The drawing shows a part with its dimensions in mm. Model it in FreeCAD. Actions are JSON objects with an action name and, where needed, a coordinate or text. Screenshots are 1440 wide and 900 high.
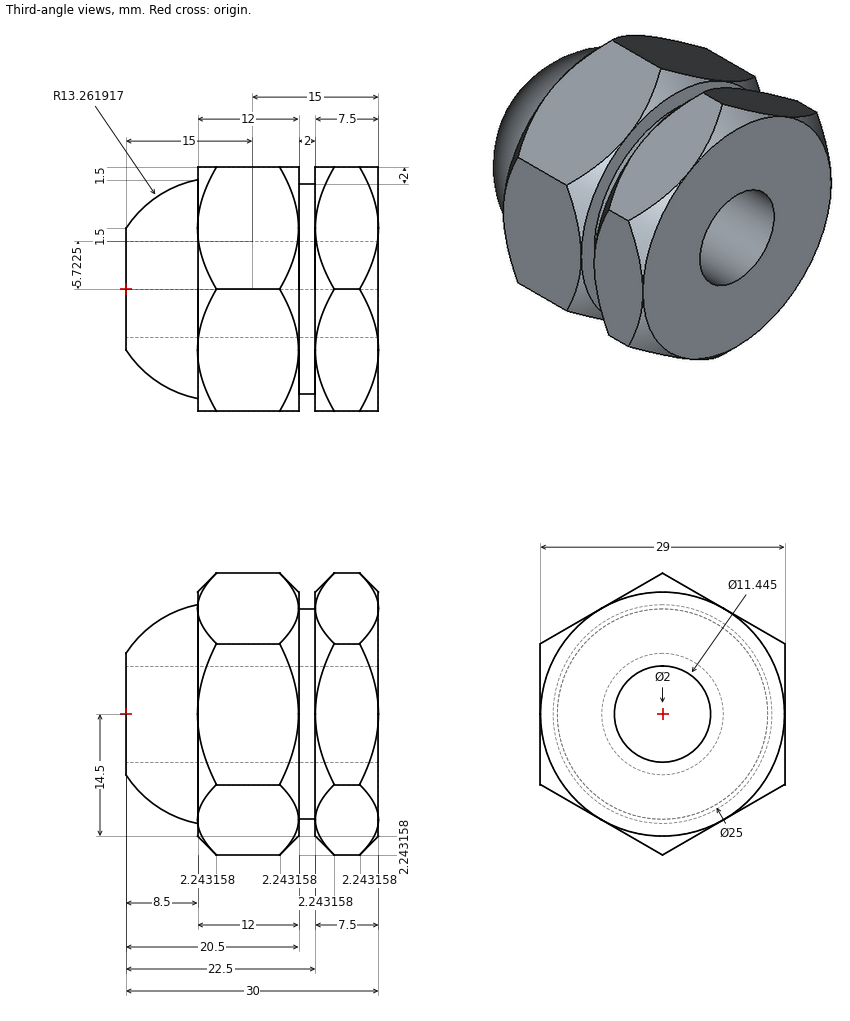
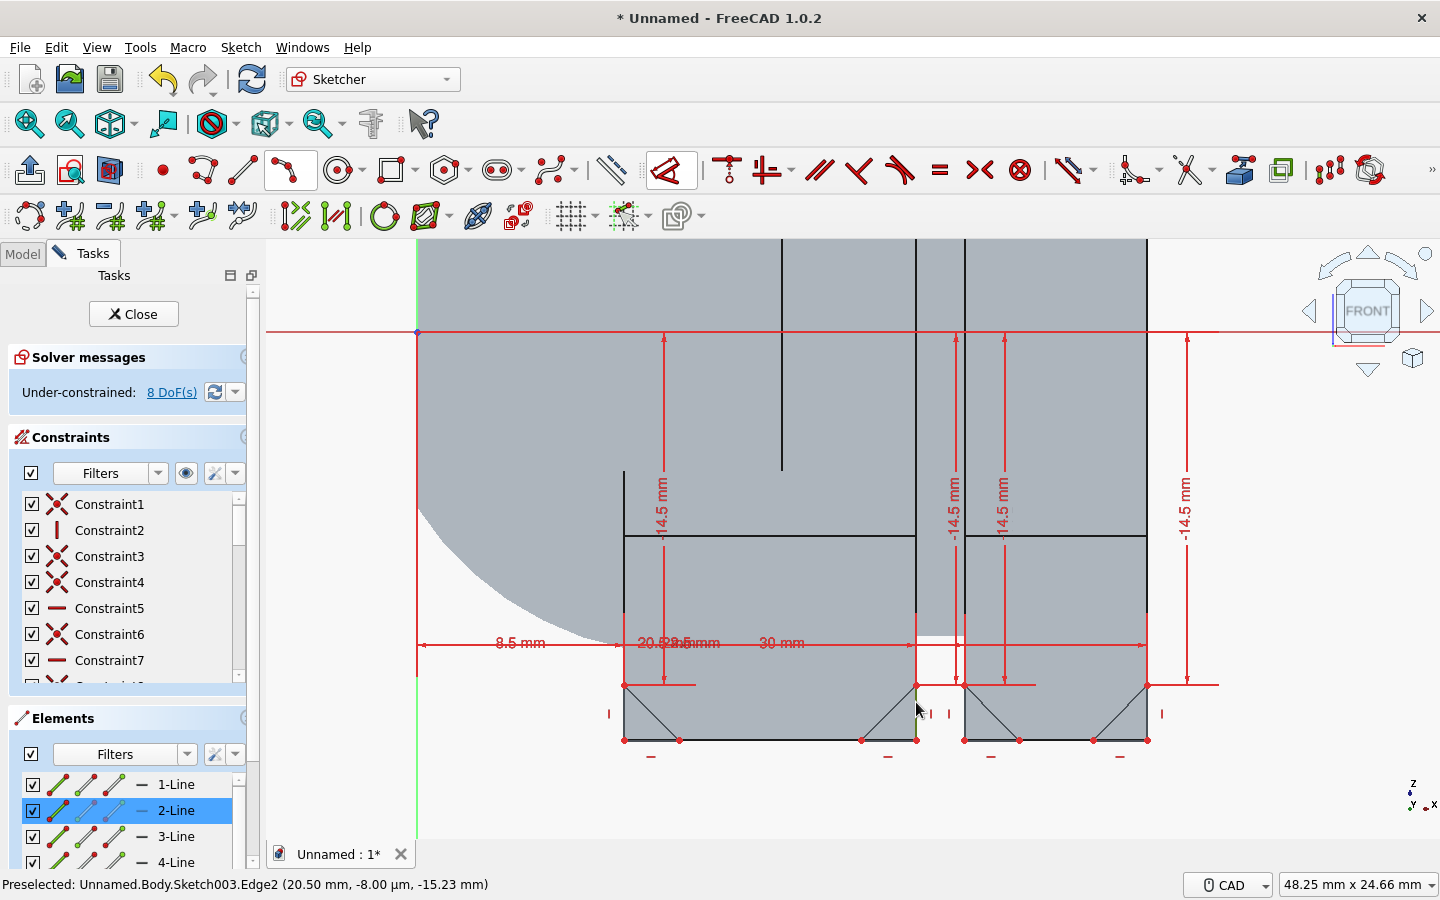
{"action": "key", "text": "i"}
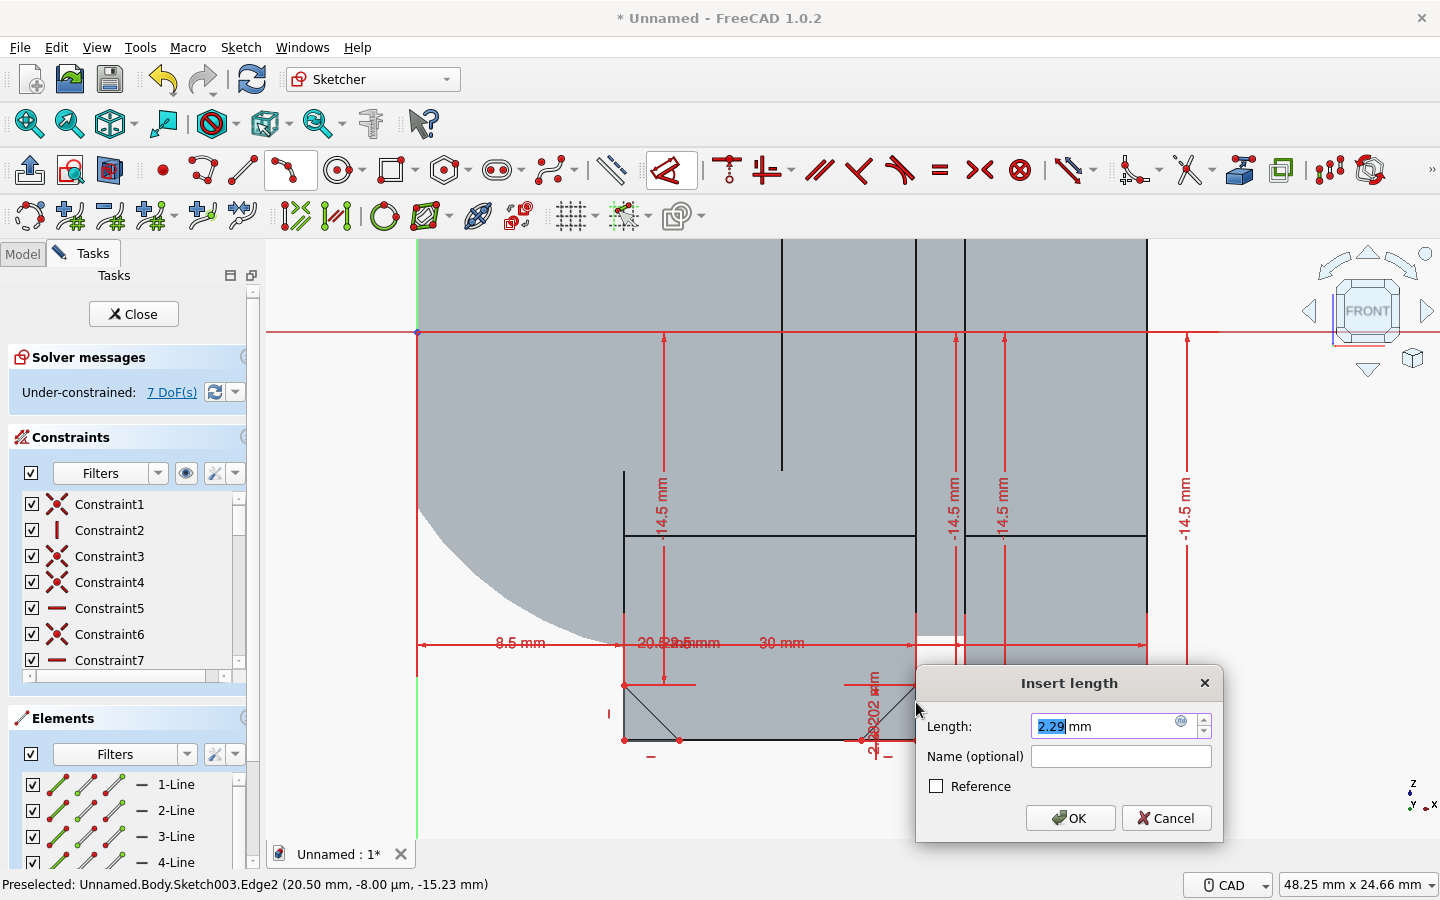
{"action": "type", "text": "2.243158"}
{"action": "key", "text": "Return"}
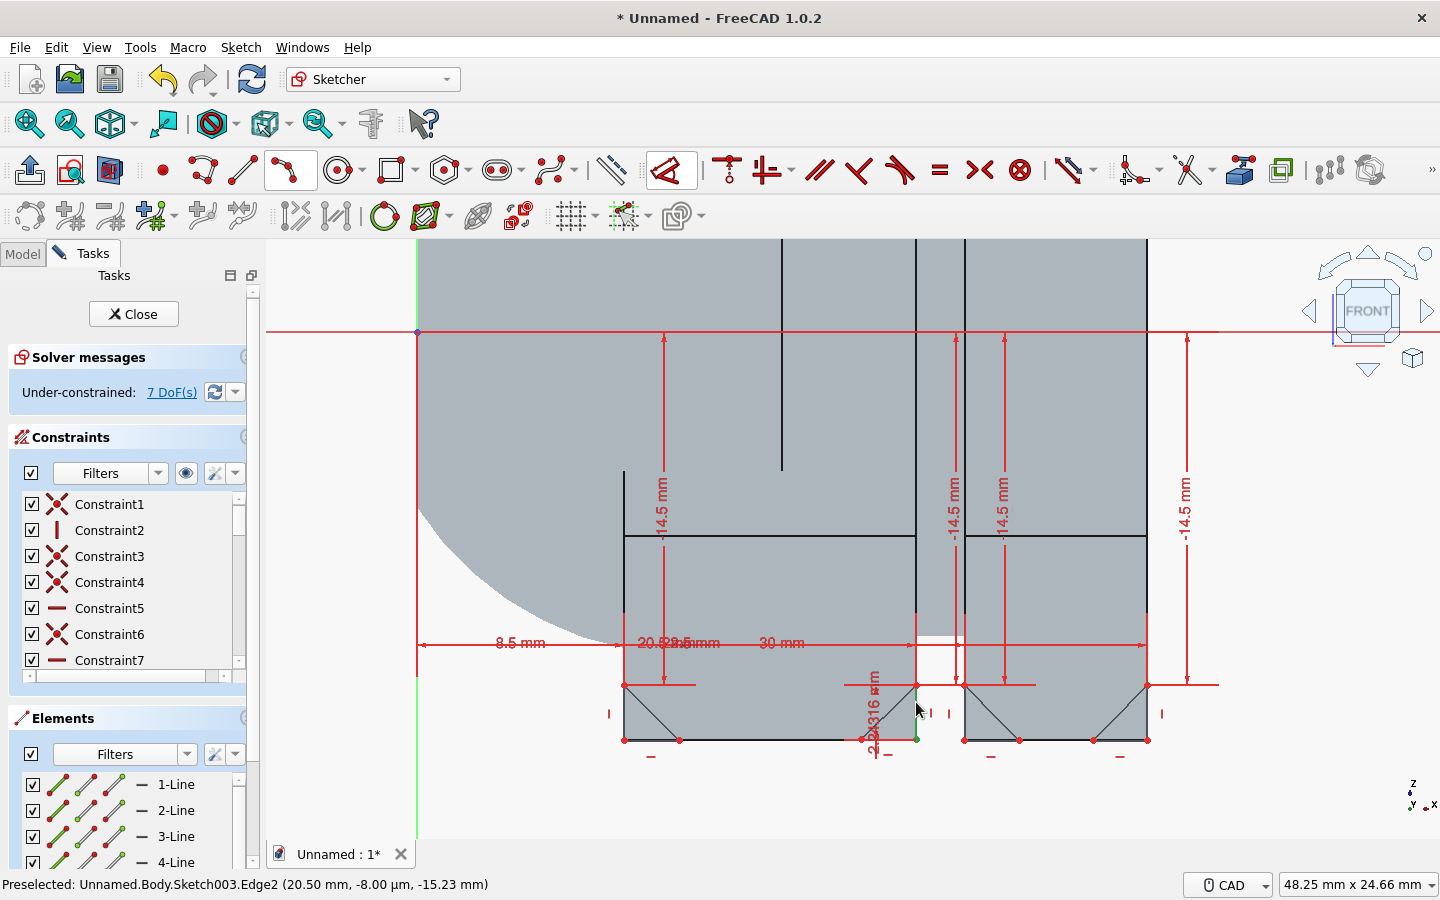
{"action": "left_click", "coordinate": [900, 740]}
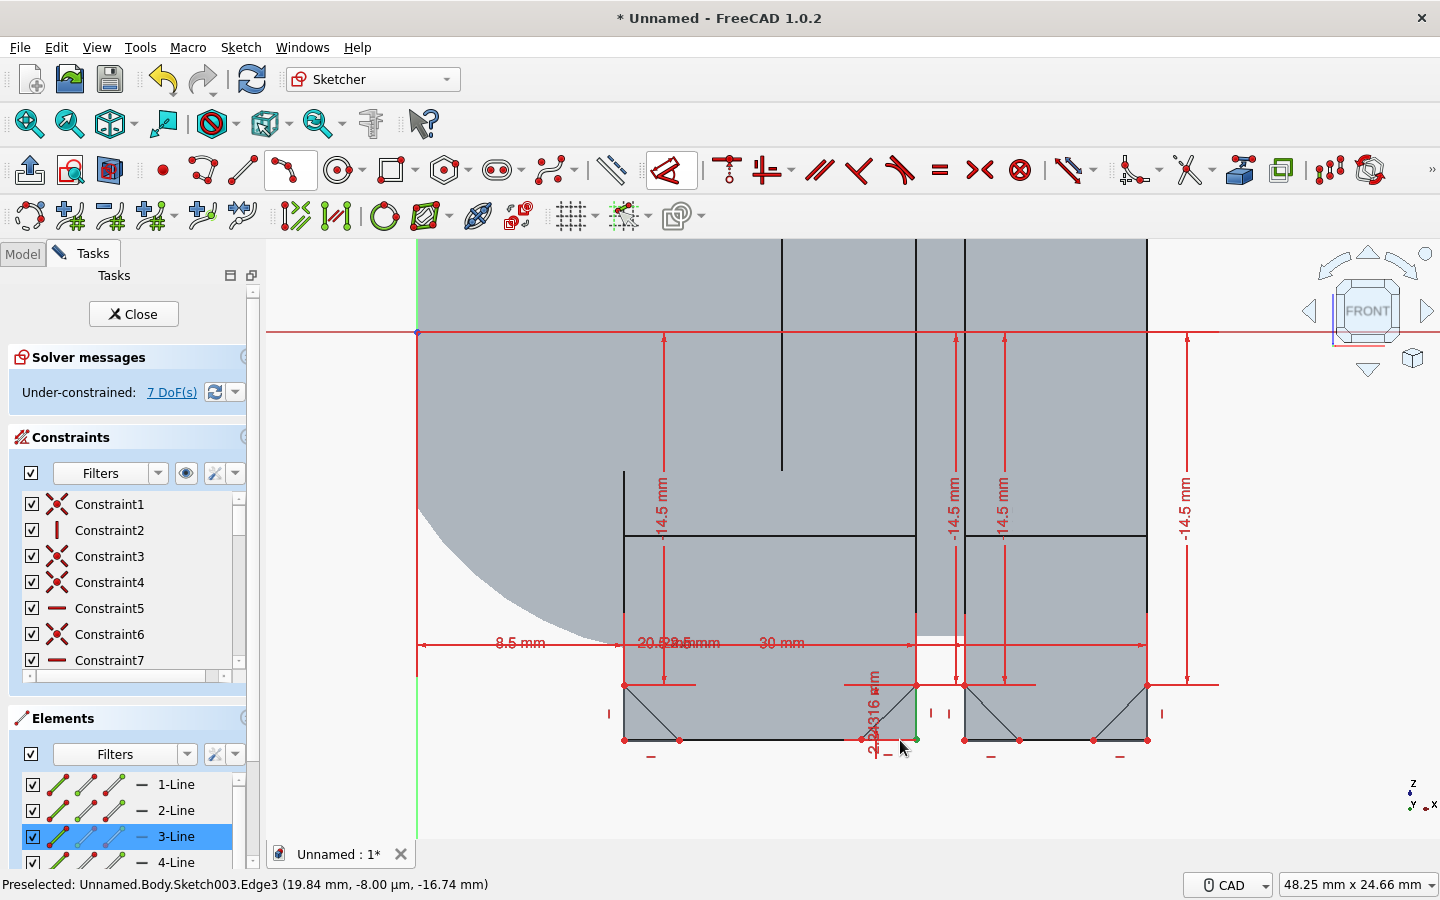
{"action": "left_click", "coordinate": [692, 170]}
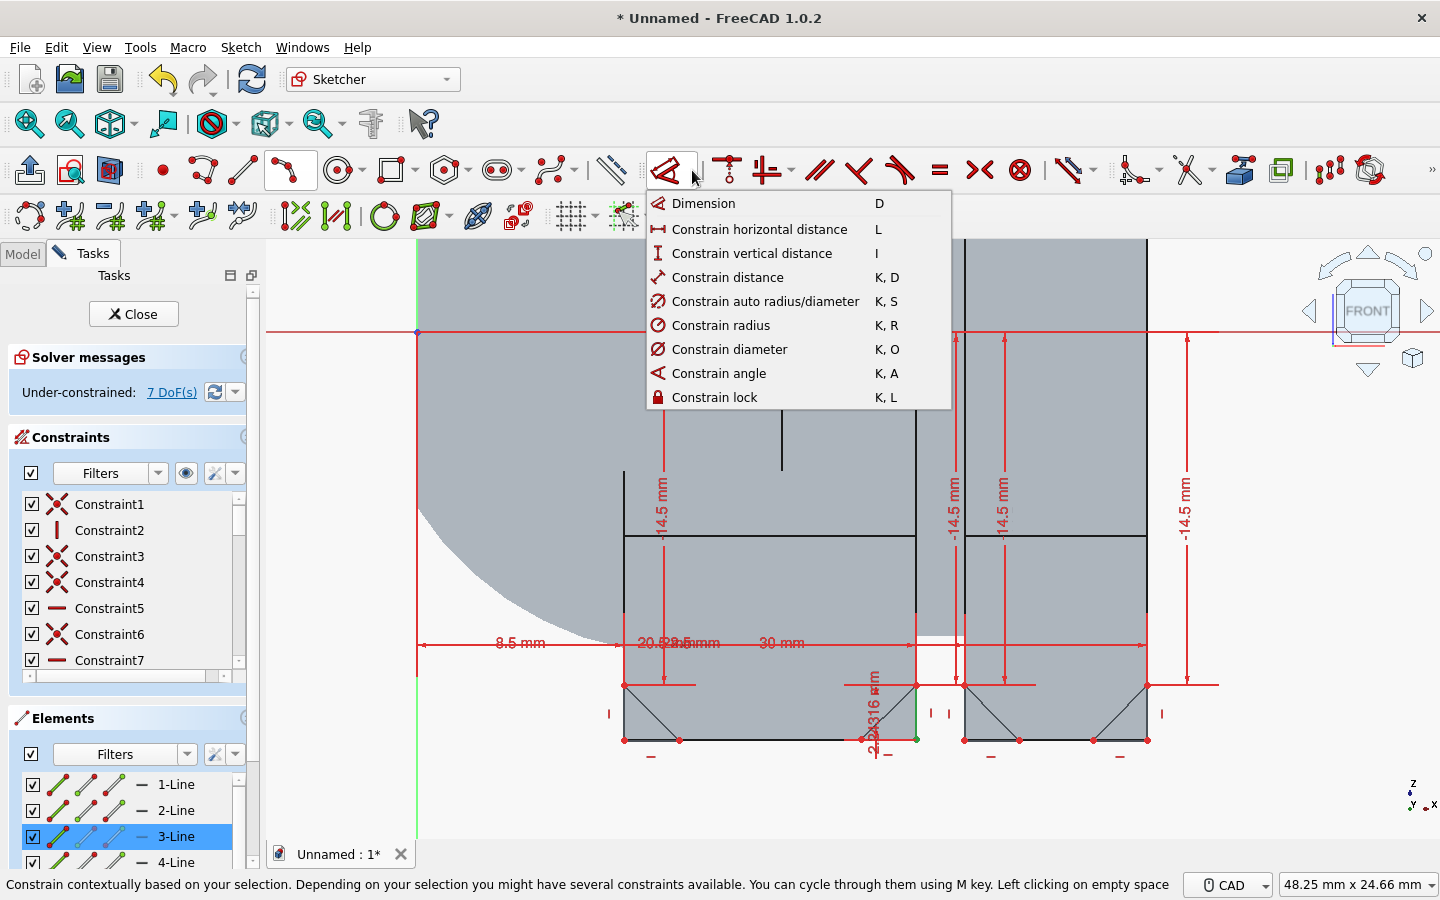
{"action": "left_click", "coordinate": [799, 229]}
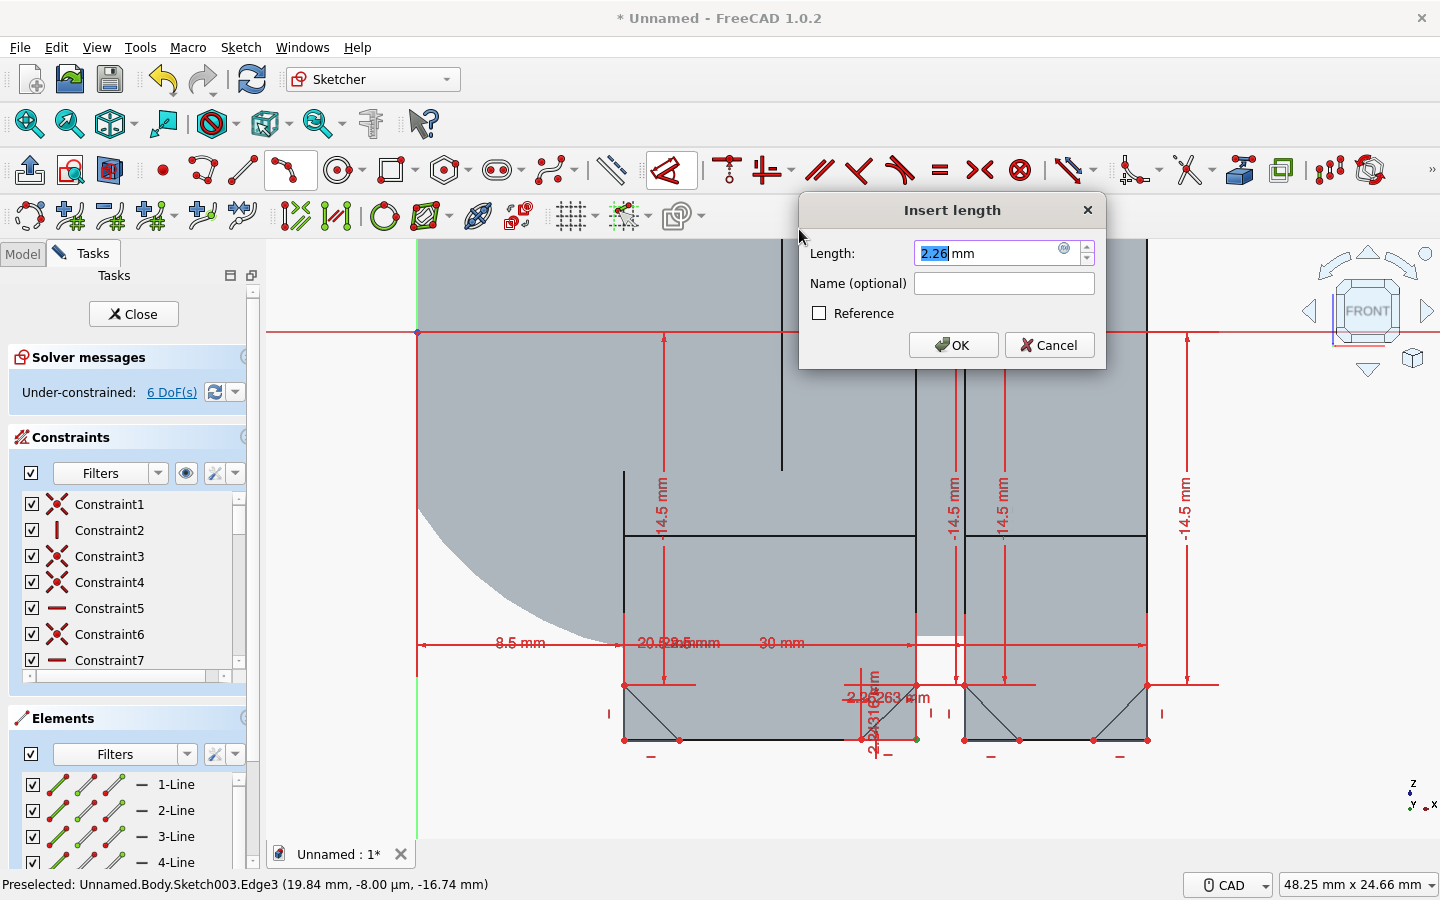
{"action": "type", "text": "2.243158"}
{"action": "key", "text": "Return"}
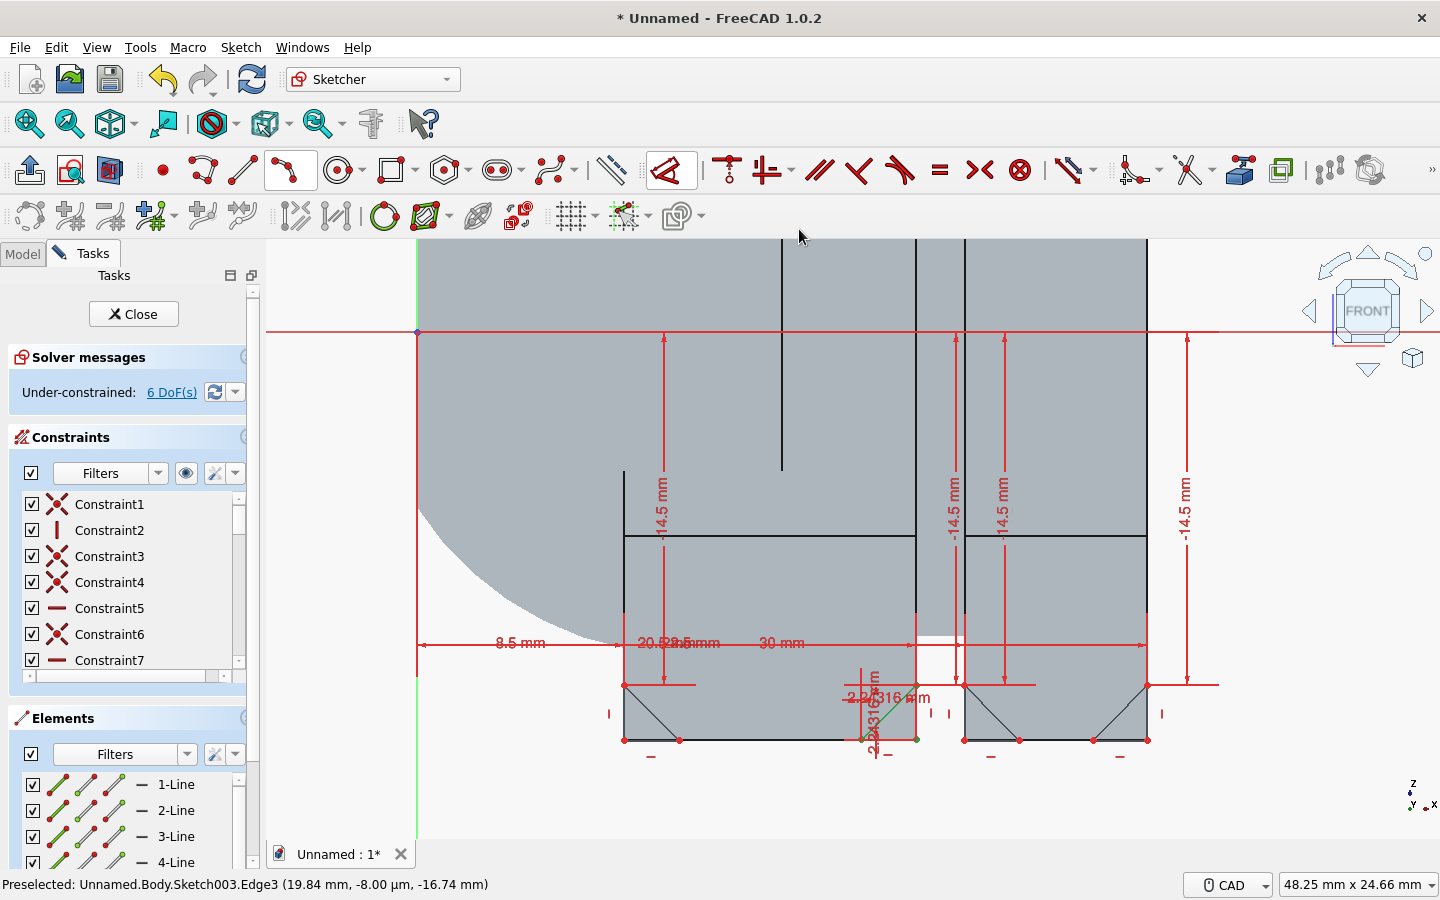
{"action": "left_click", "coordinate": [1003, 741]}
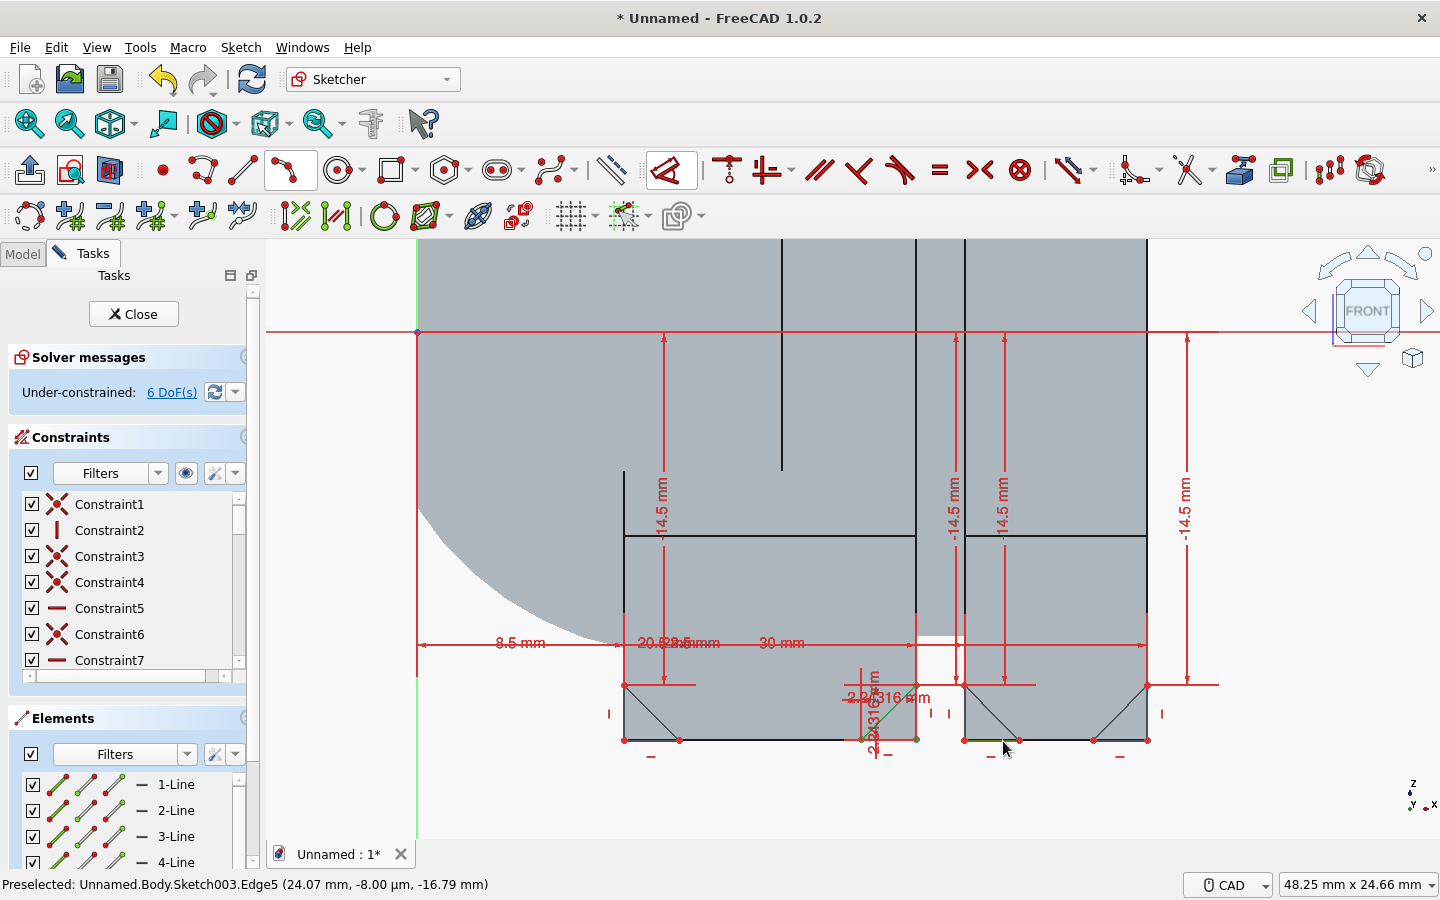
{"action": "left_click", "coordinate": [692, 170]}